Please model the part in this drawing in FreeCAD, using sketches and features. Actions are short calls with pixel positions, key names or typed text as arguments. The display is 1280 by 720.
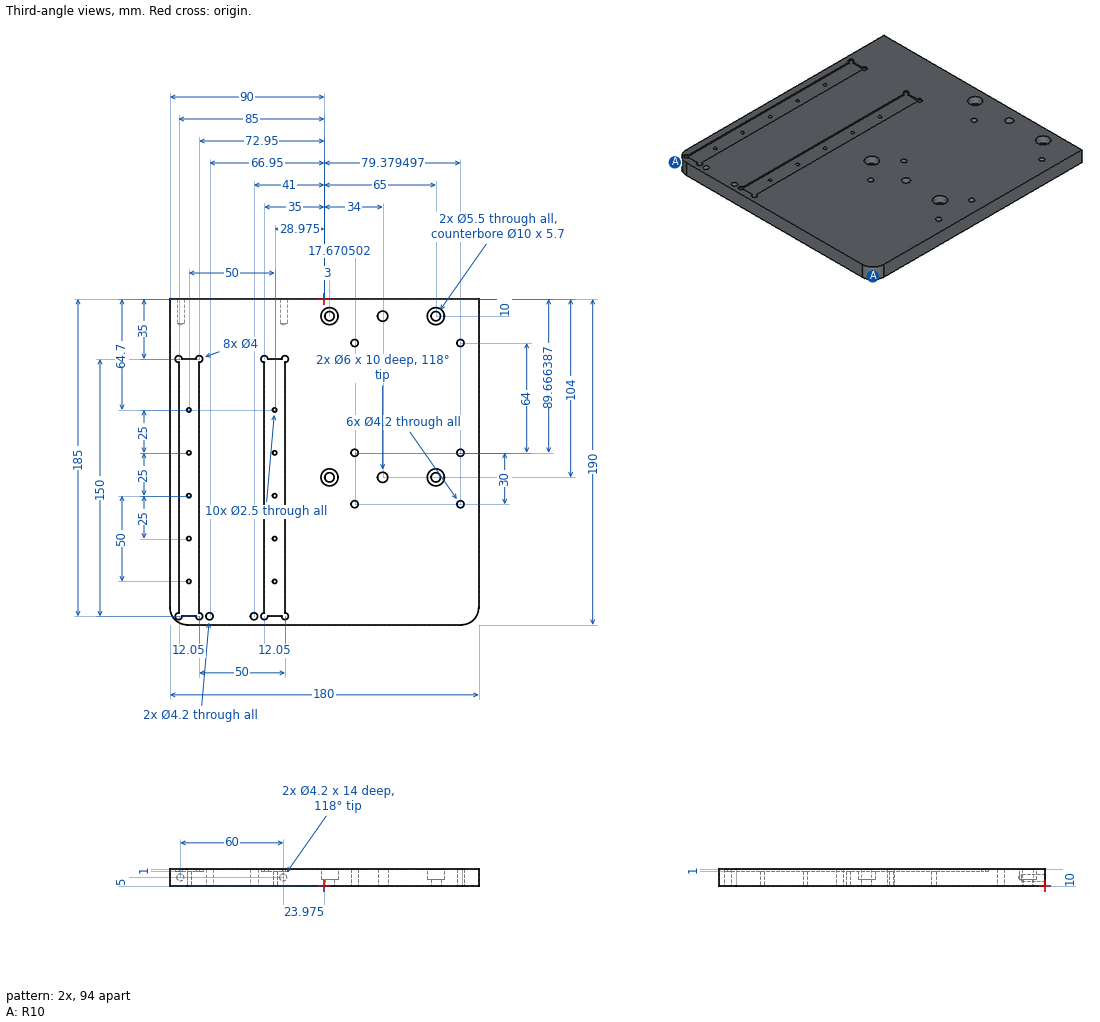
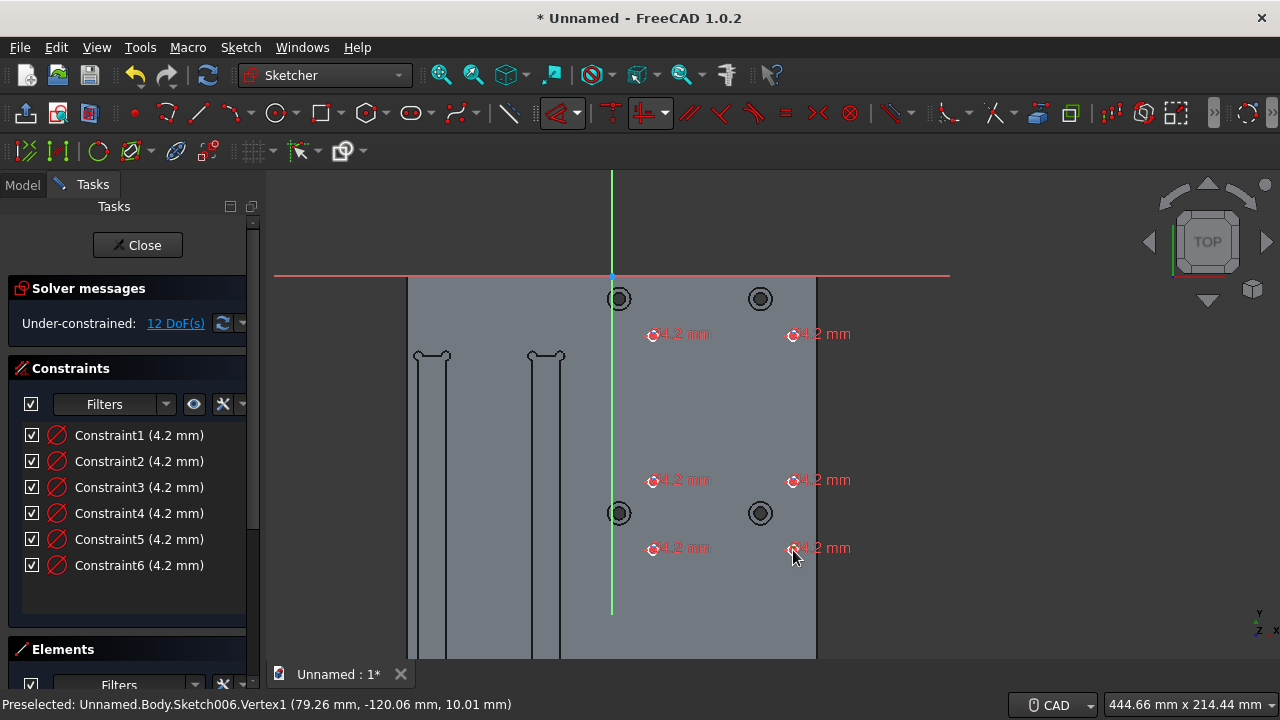
click(653, 550)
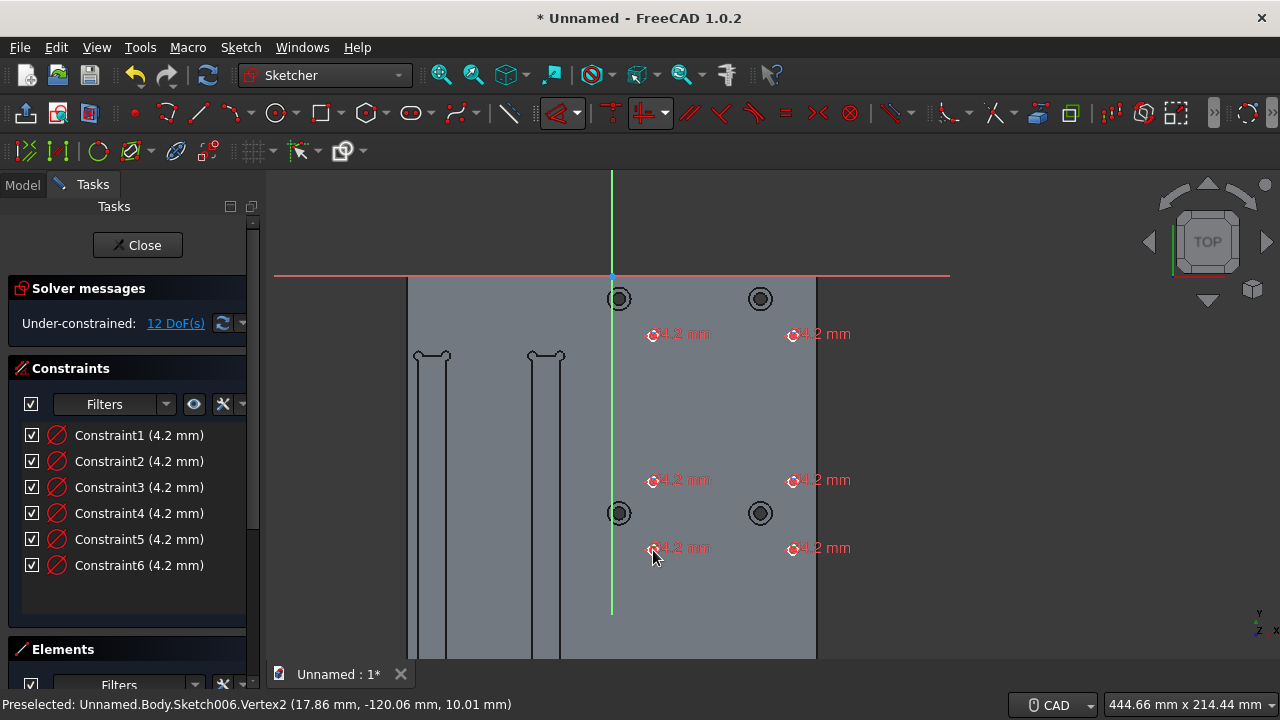
key(h)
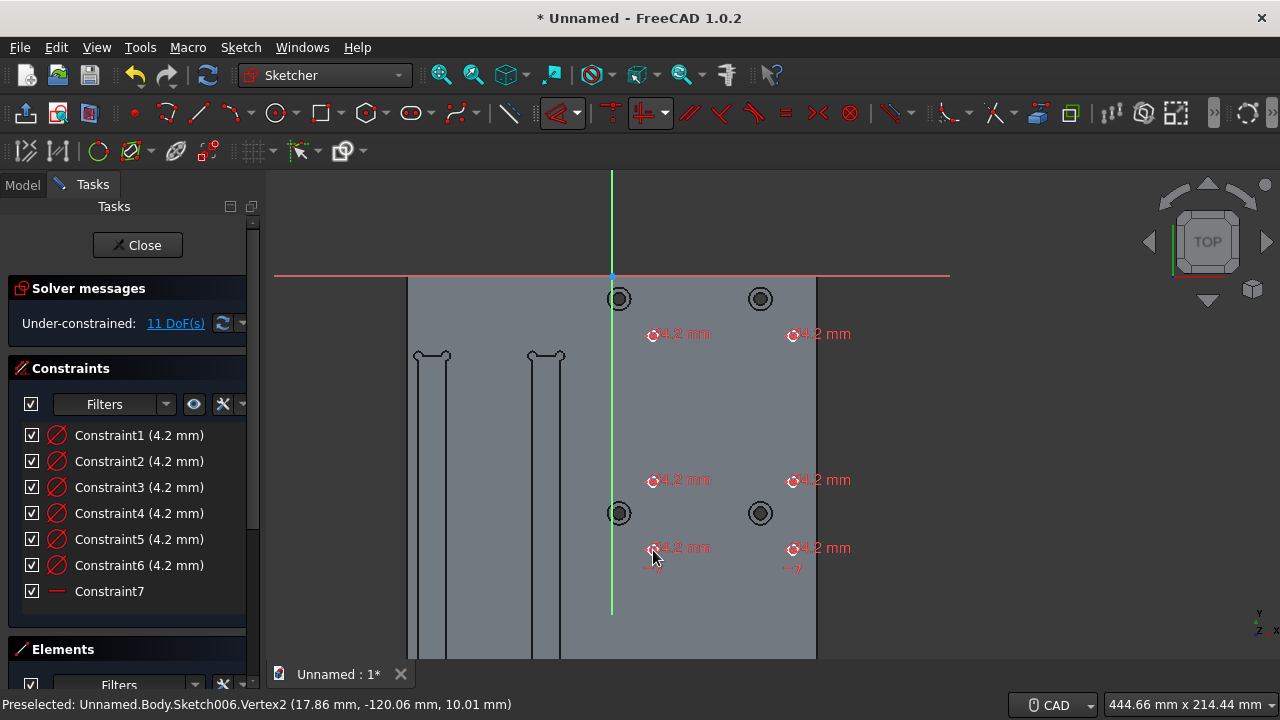
click(653, 550)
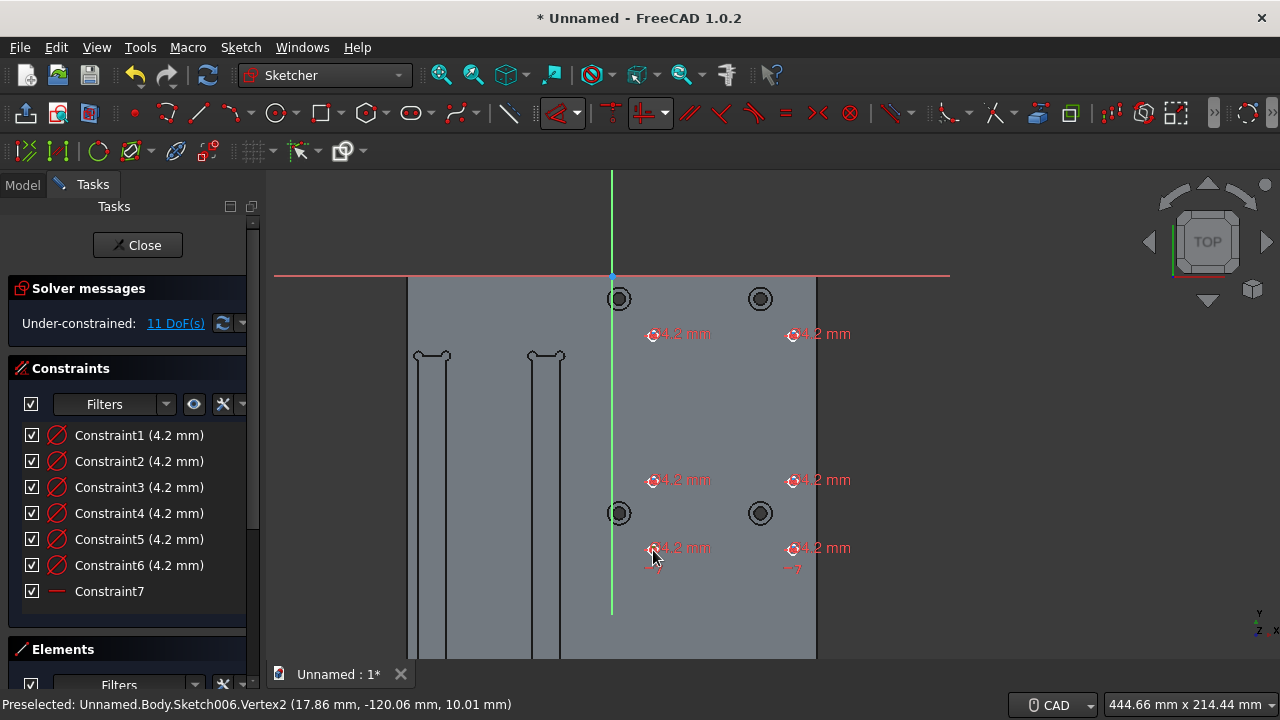
click(653, 482)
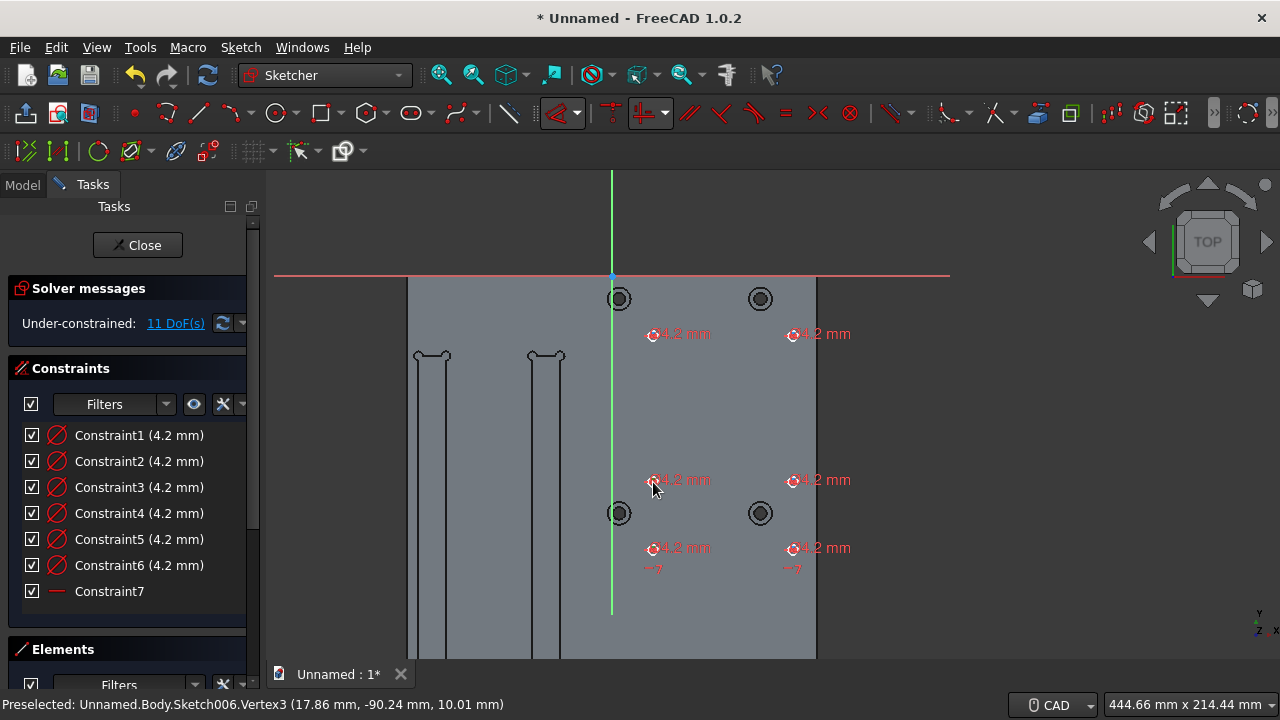
click(668, 114)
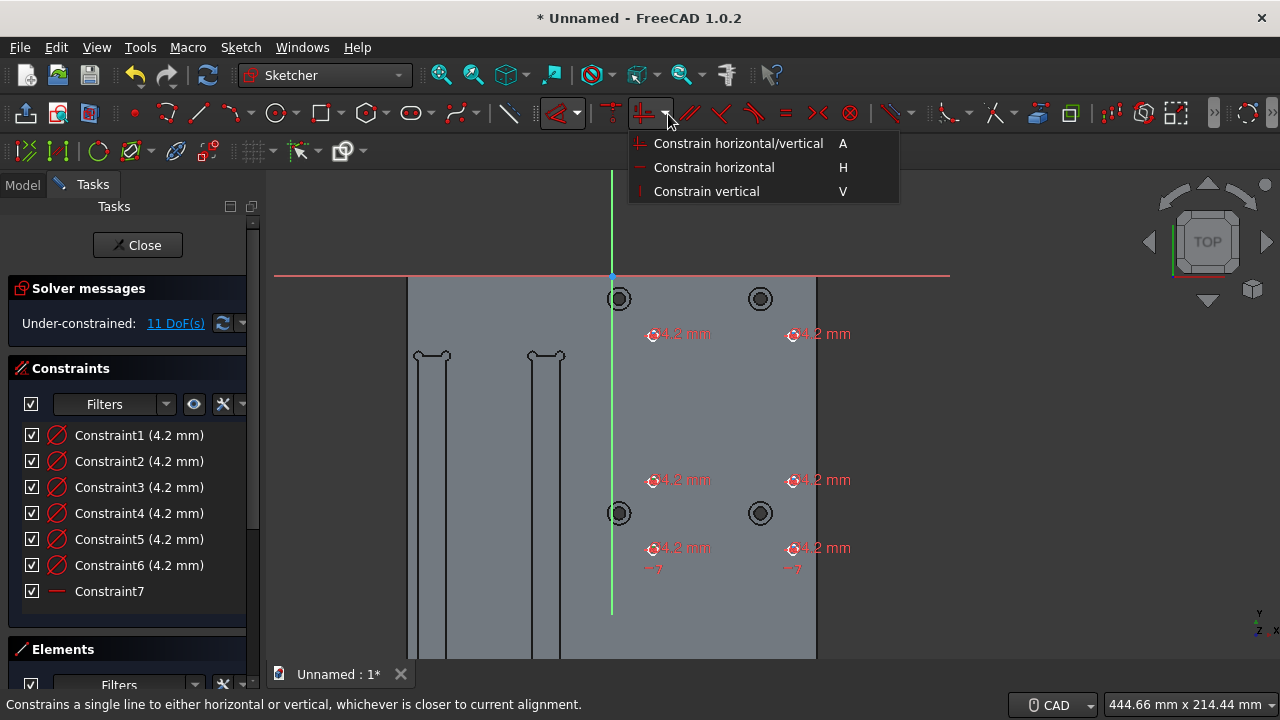
click(764, 191)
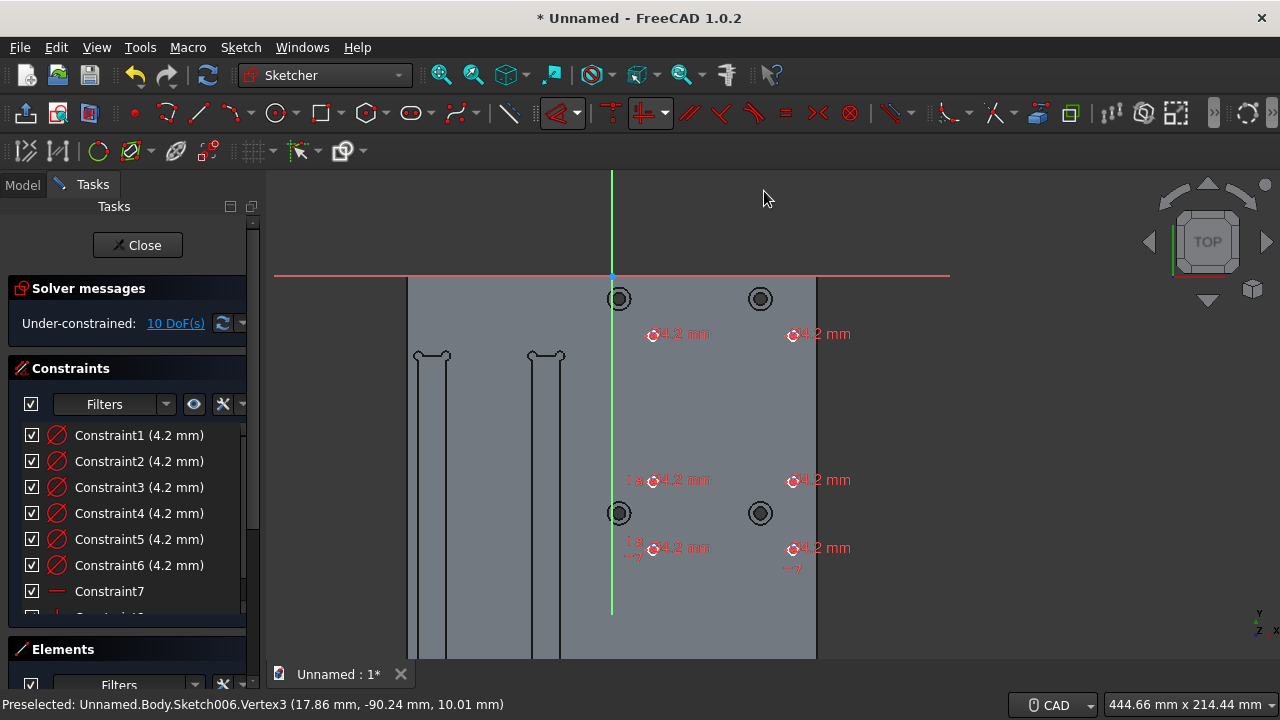
click(793, 550)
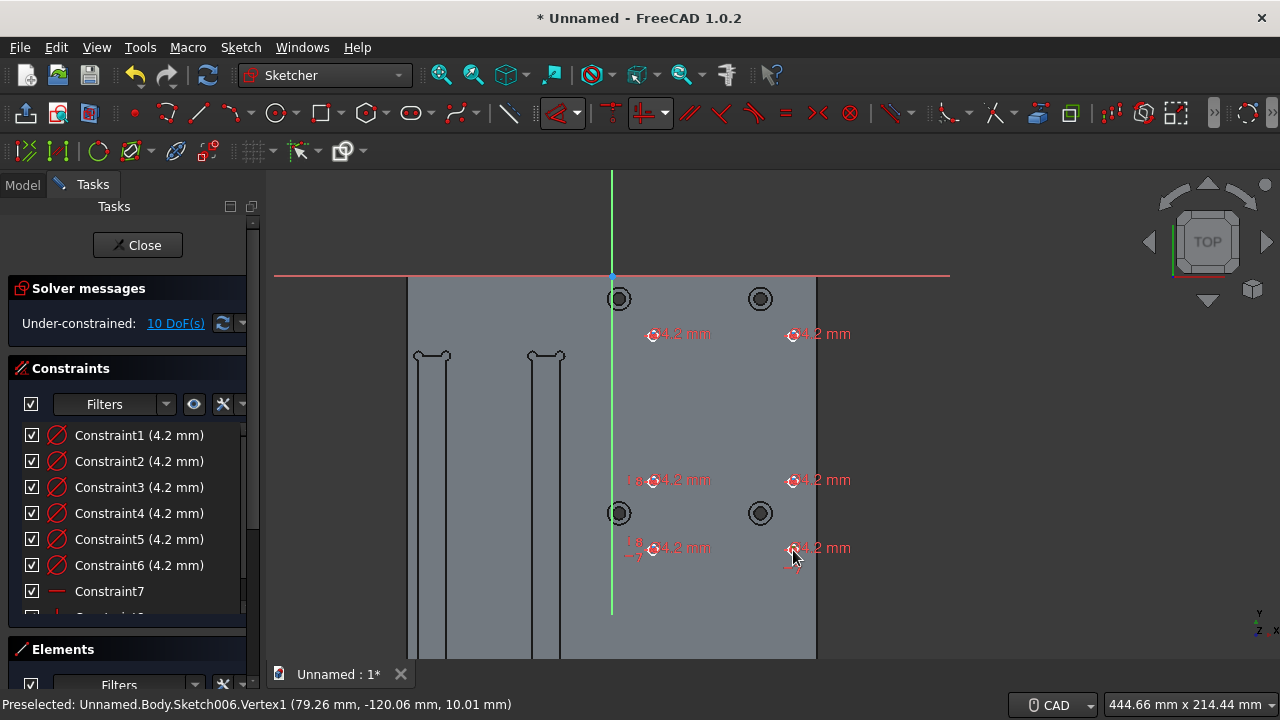
click(793, 482)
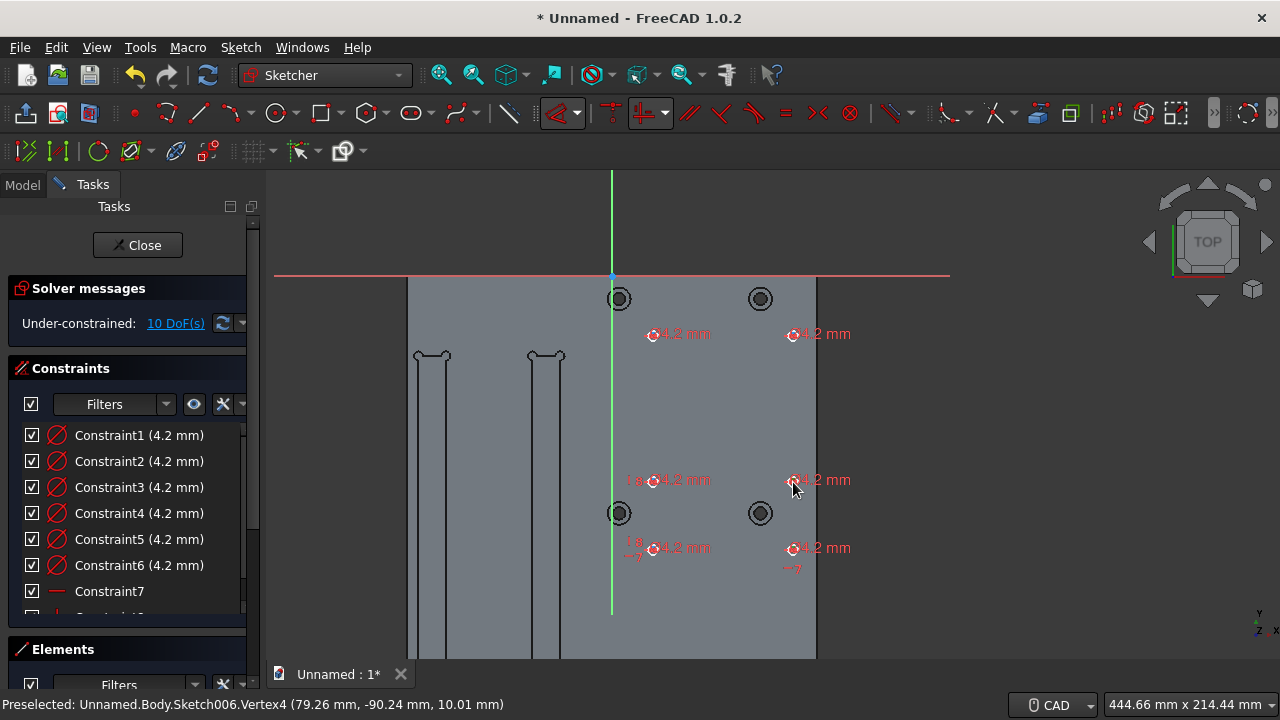
click(668, 114)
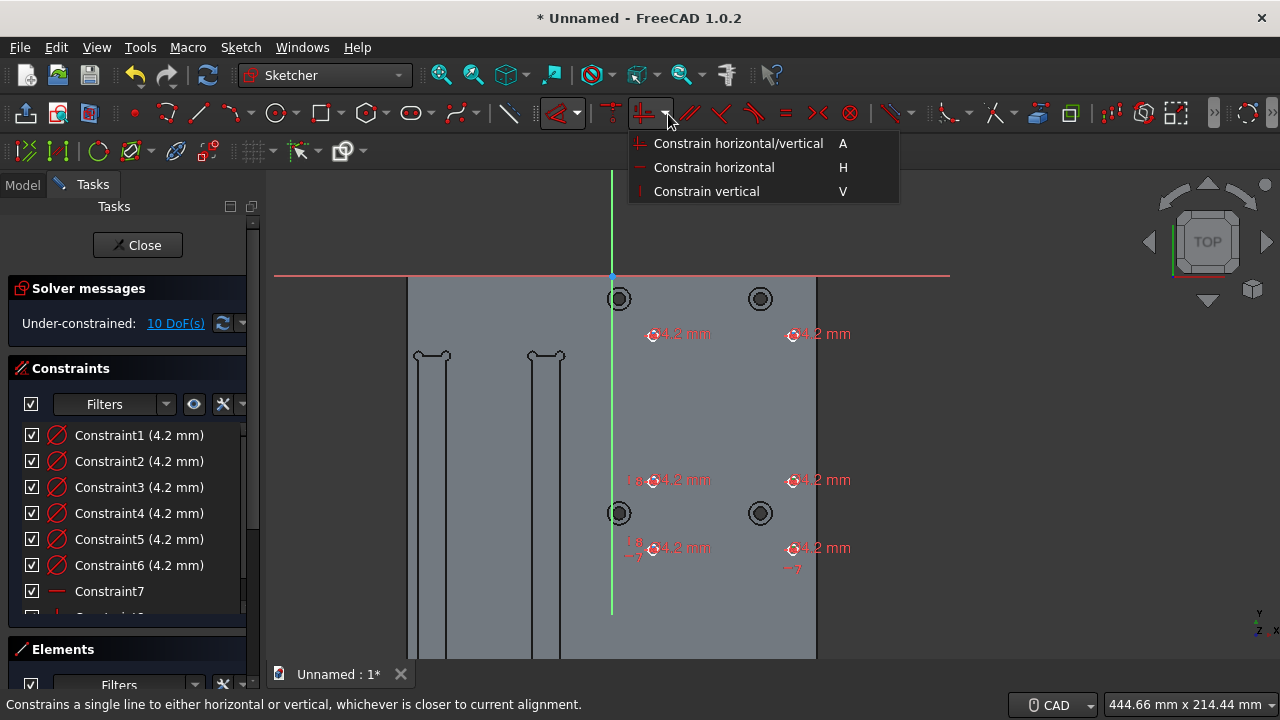
click(764, 191)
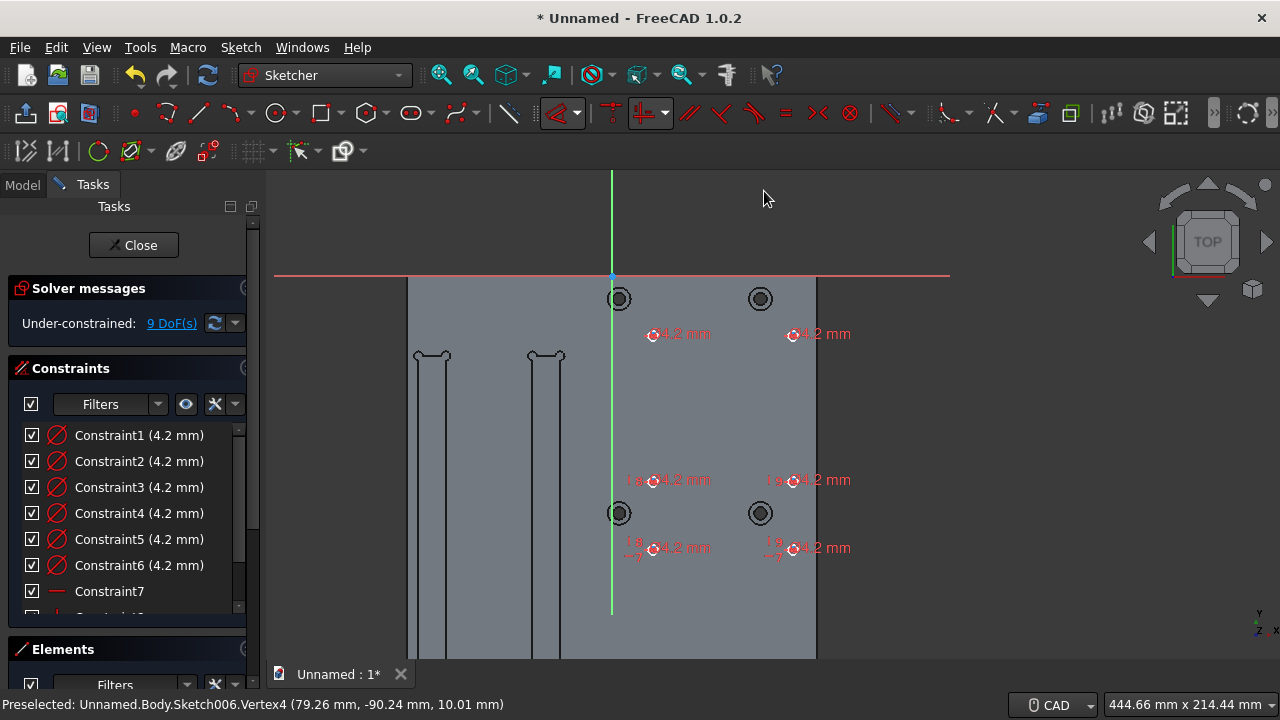
click(653, 482)